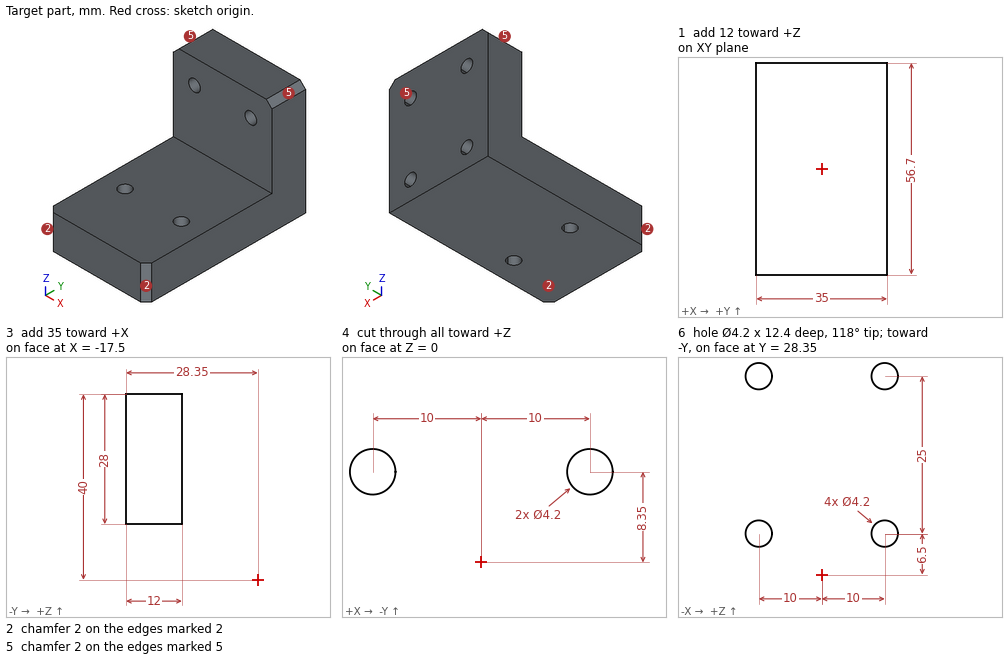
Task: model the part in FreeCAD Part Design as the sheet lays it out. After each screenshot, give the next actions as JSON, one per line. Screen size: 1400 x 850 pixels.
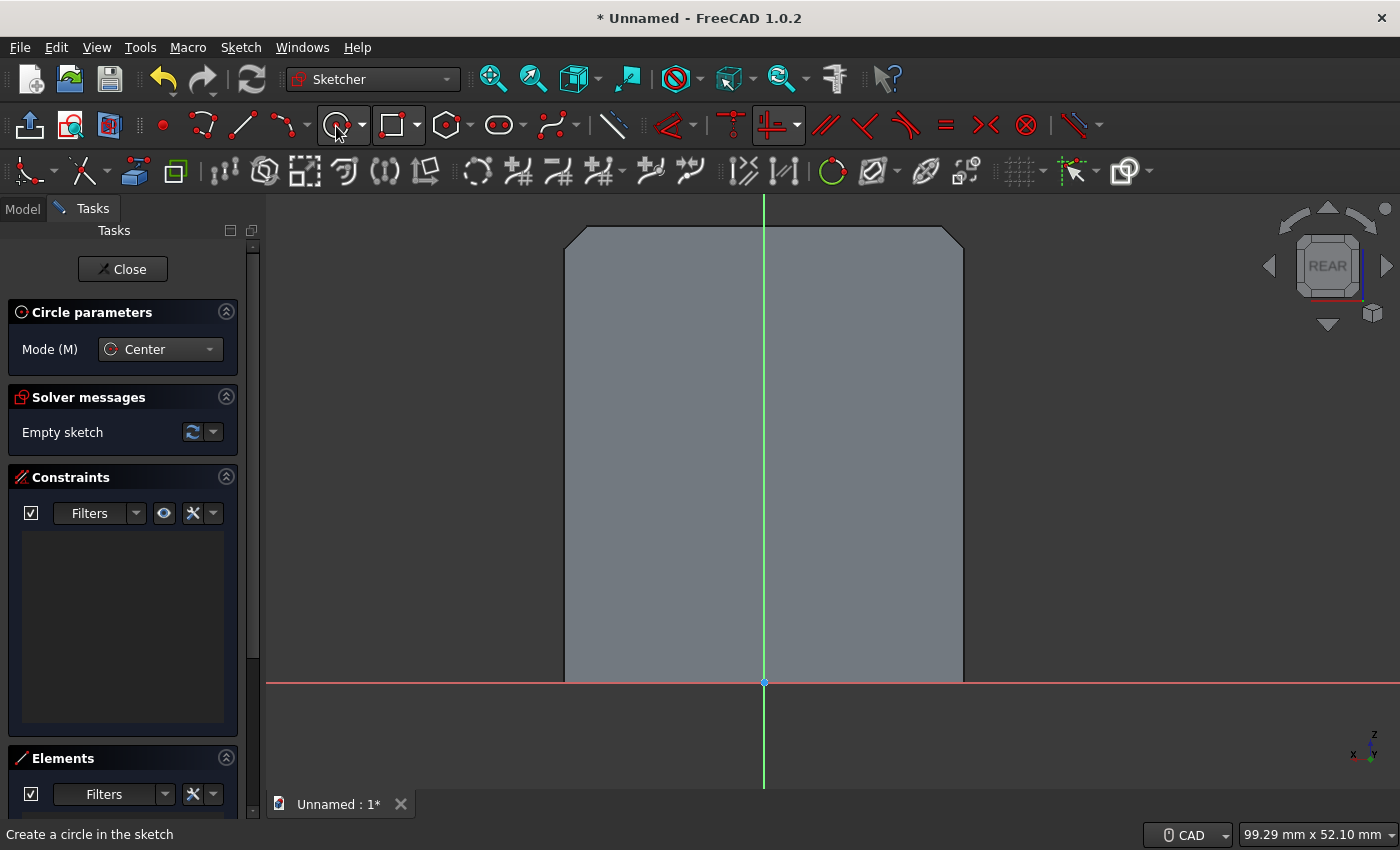
{"action": "left_click", "coordinate": [879, 609]}
{"action": "left_click", "coordinate": [896, 592]}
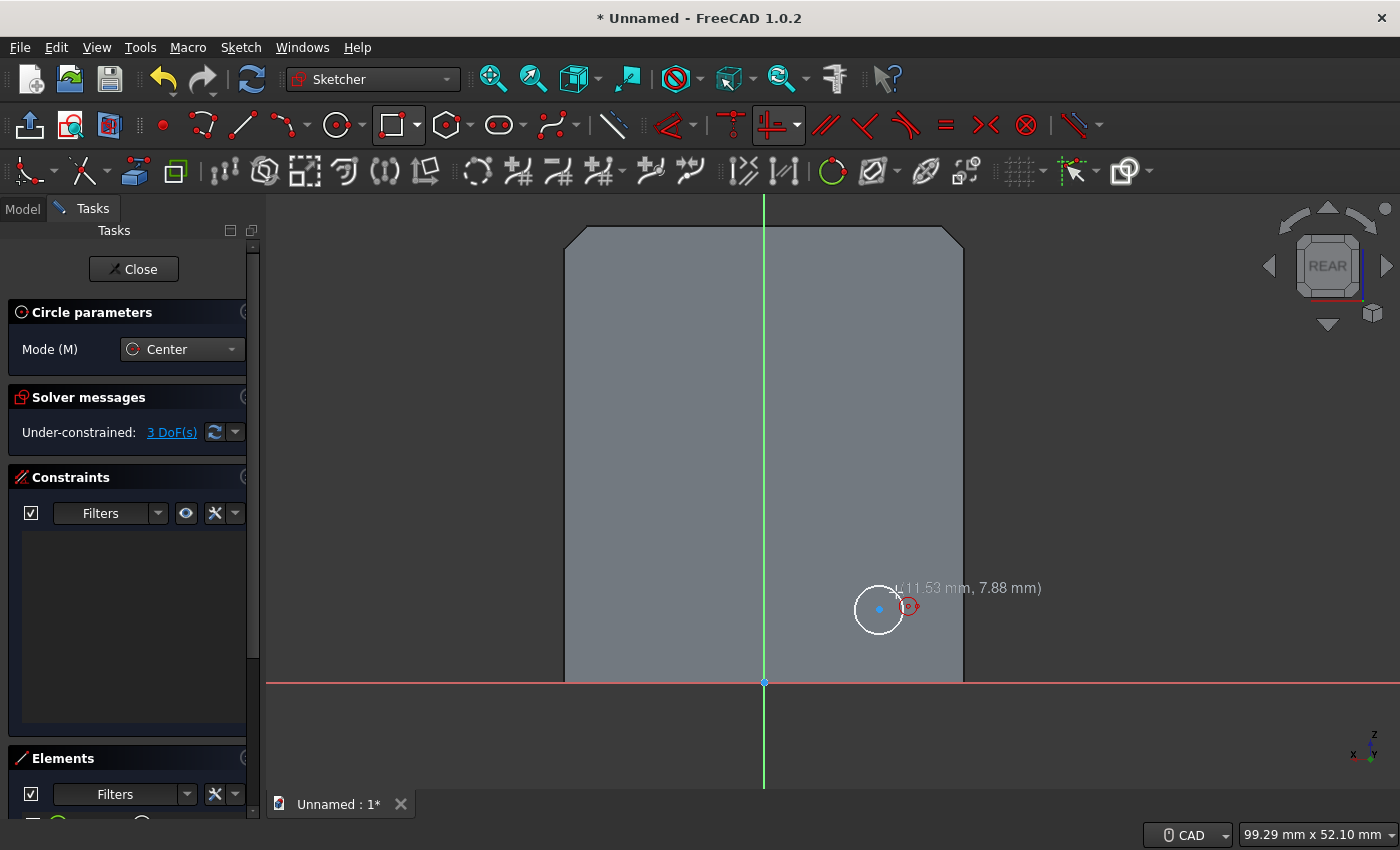
{"action": "left_click", "coordinate": [650, 609]}
{"action": "left_click", "coordinate": [667, 592]}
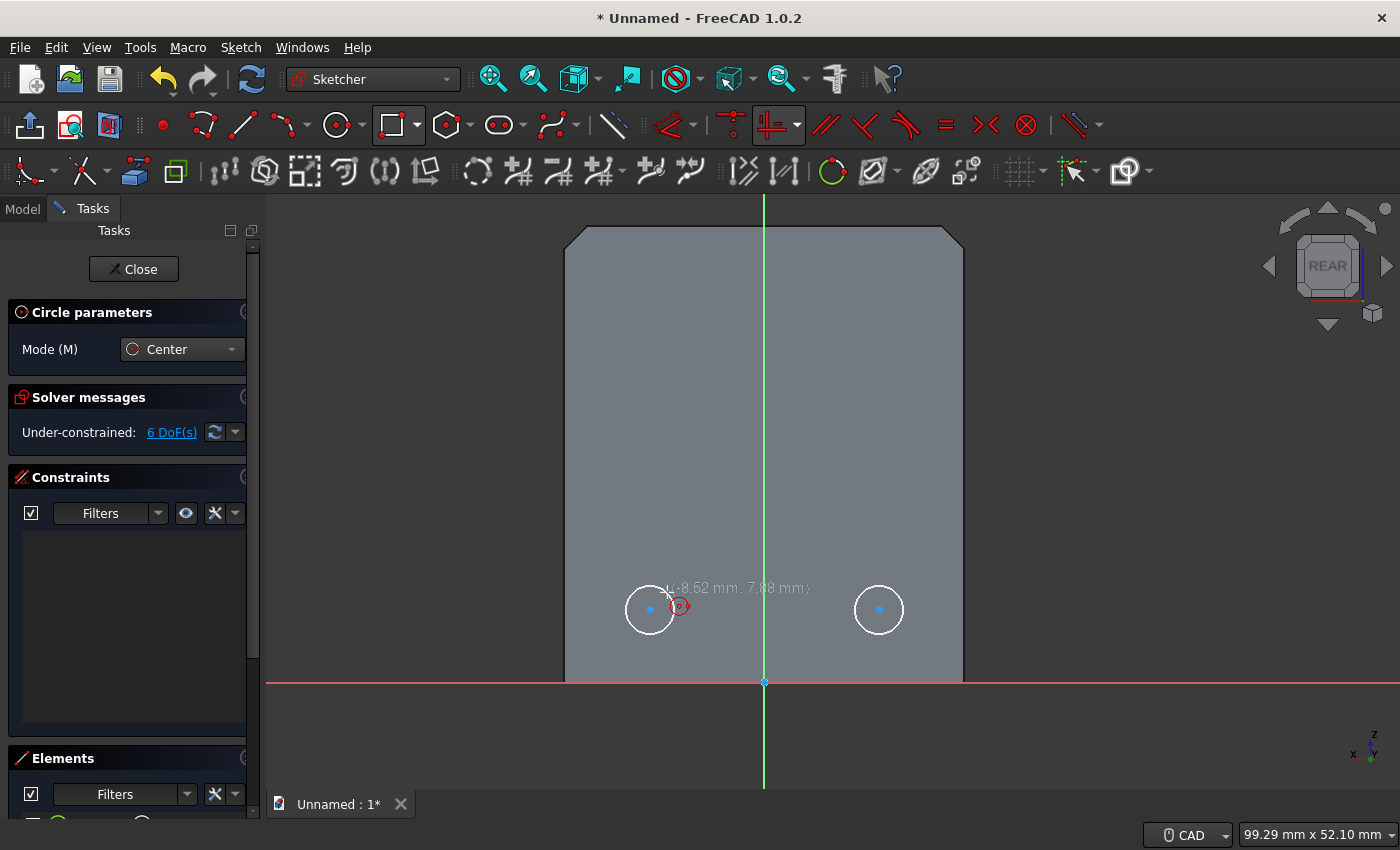
{"action": "left_click", "coordinate": [879, 323]}
{"action": "left_click", "coordinate": [896, 306]}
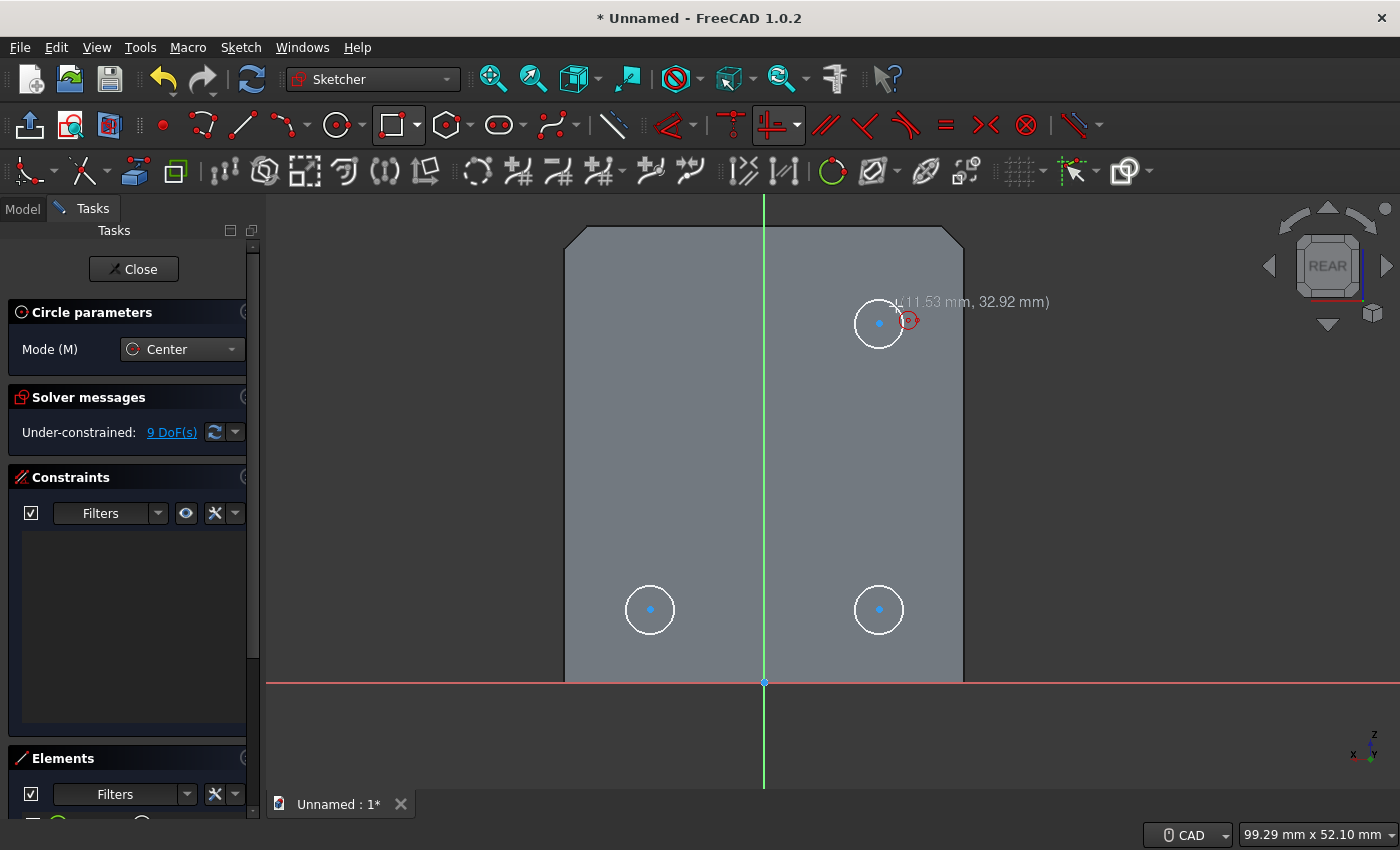
{"action": "left_click", "coordinate": [650, 323]}
{"action": "left_click", "coordinate": [667, 306]}
{"action": "key", "text": "Escape"}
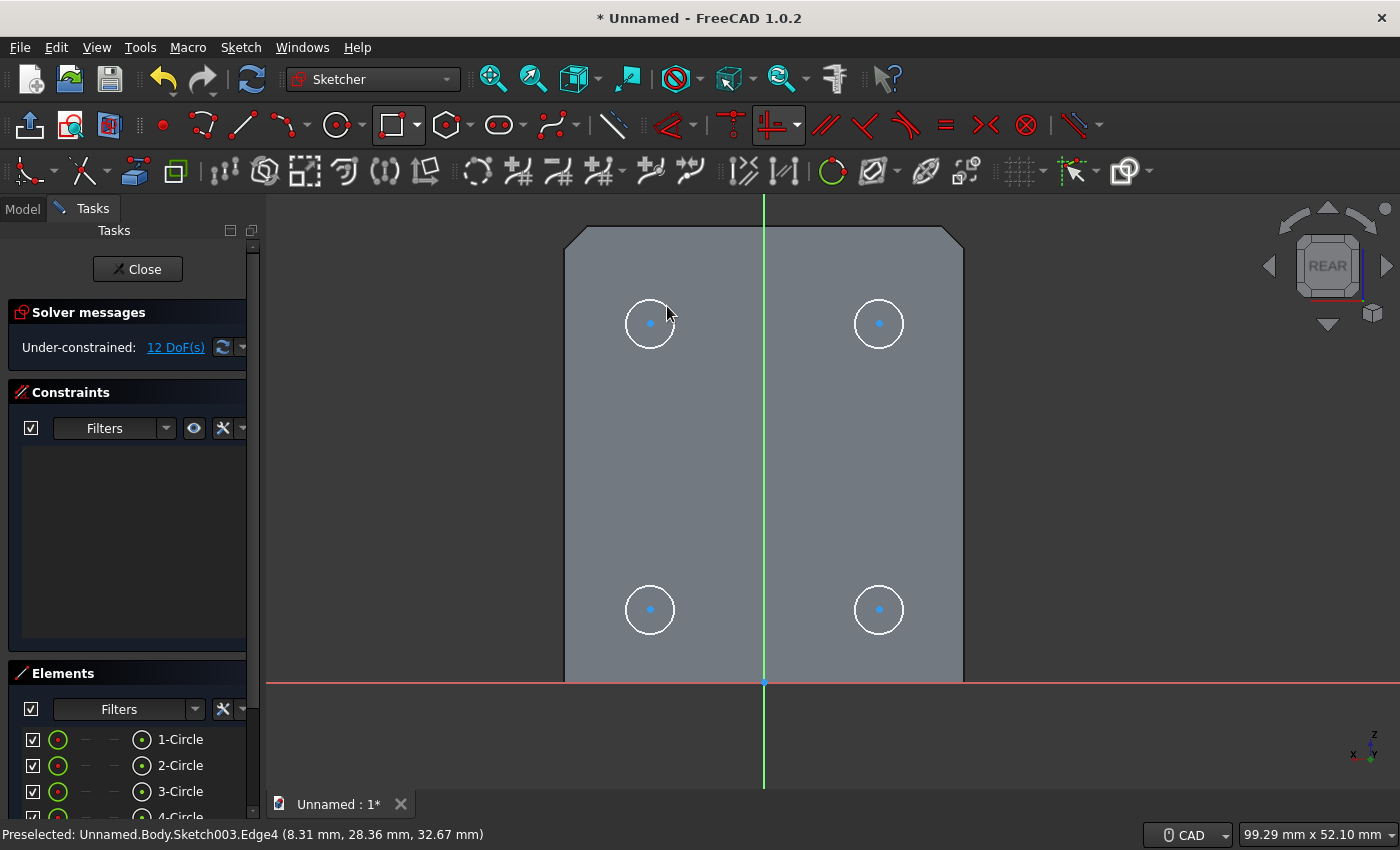
{"action": "left_click", "coordinate": [896, 593]}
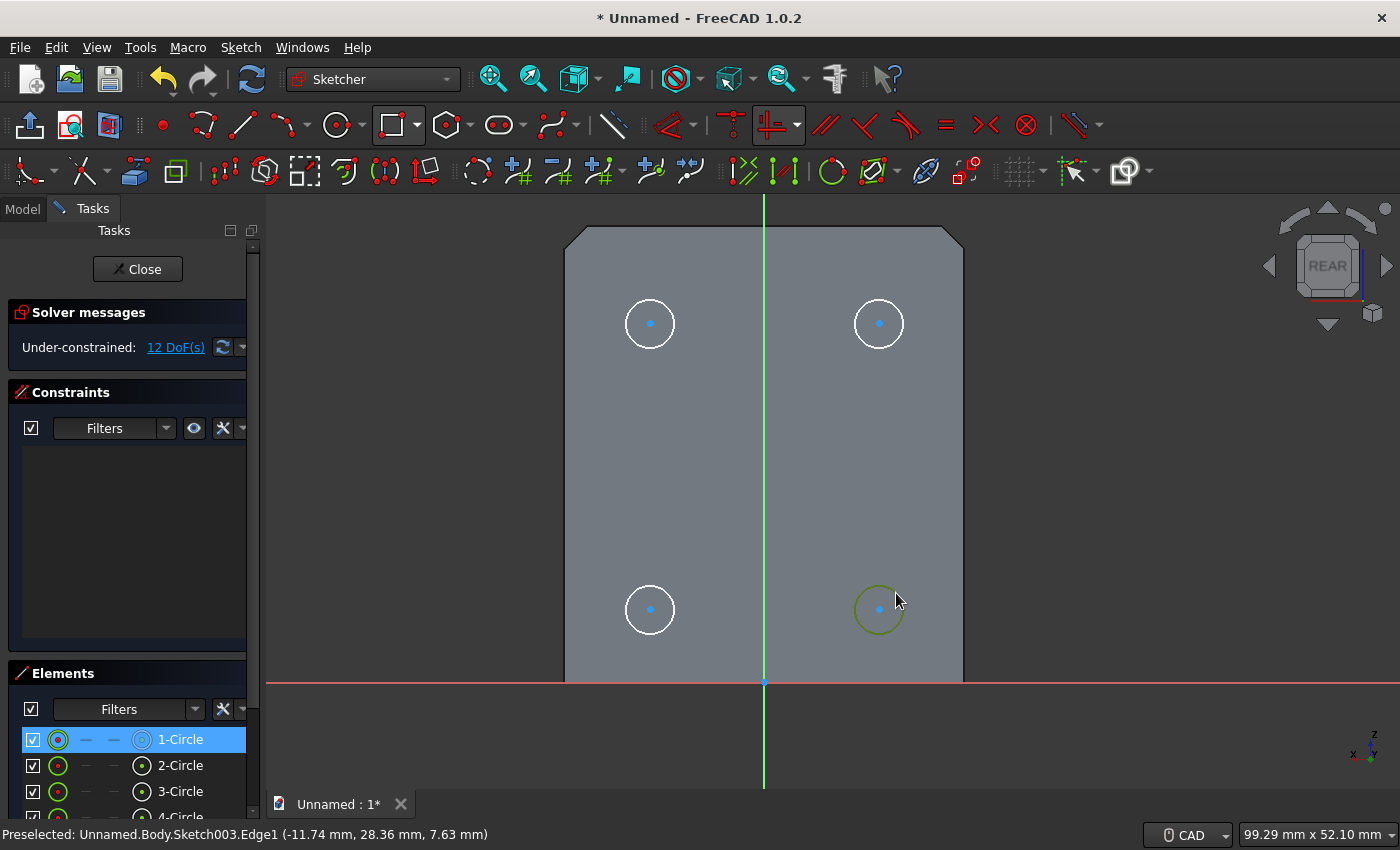
{"action": "left_click", "coordinate": [667, 593]}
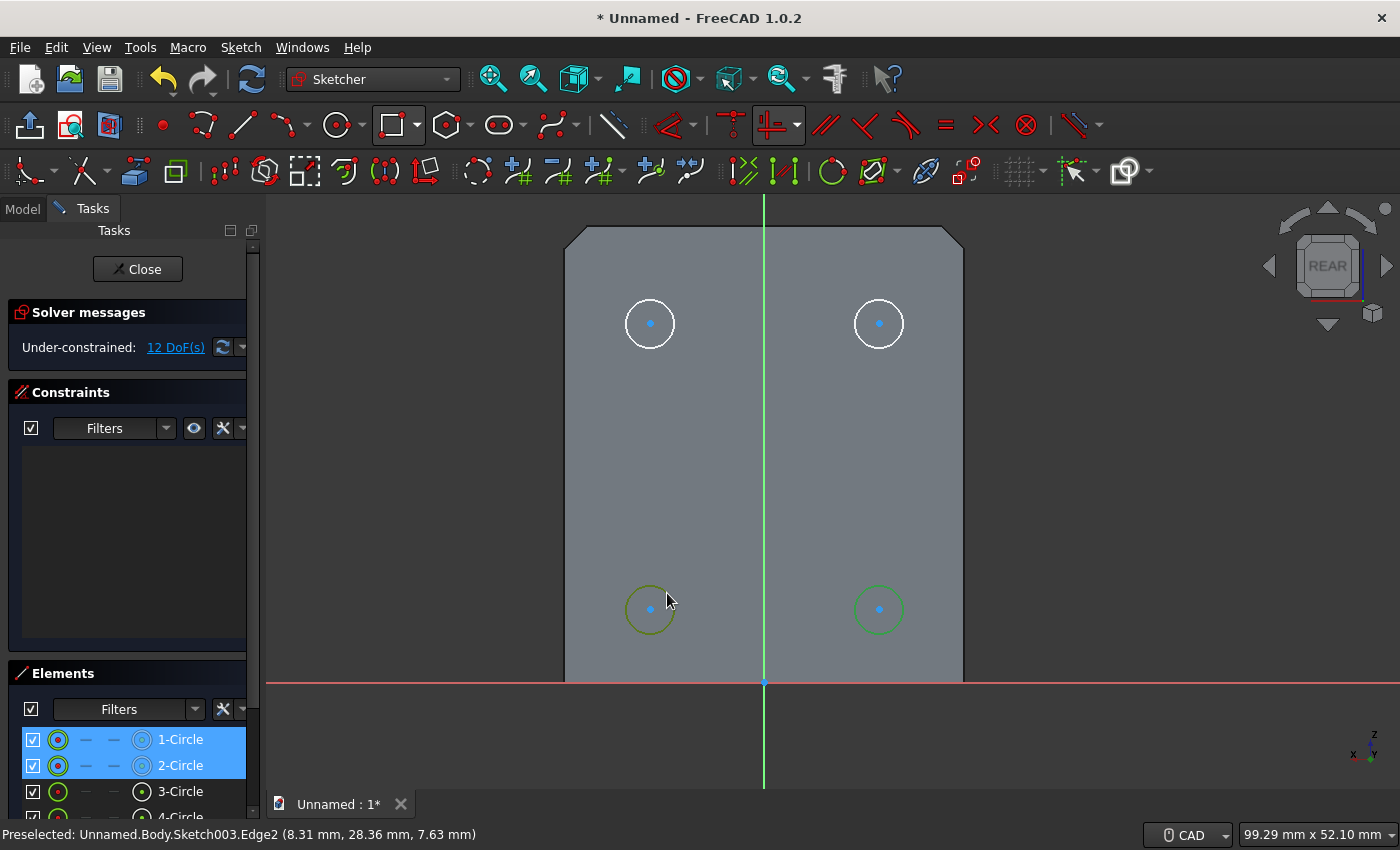
{"action": "left_click", "coordinate": [896, 307]}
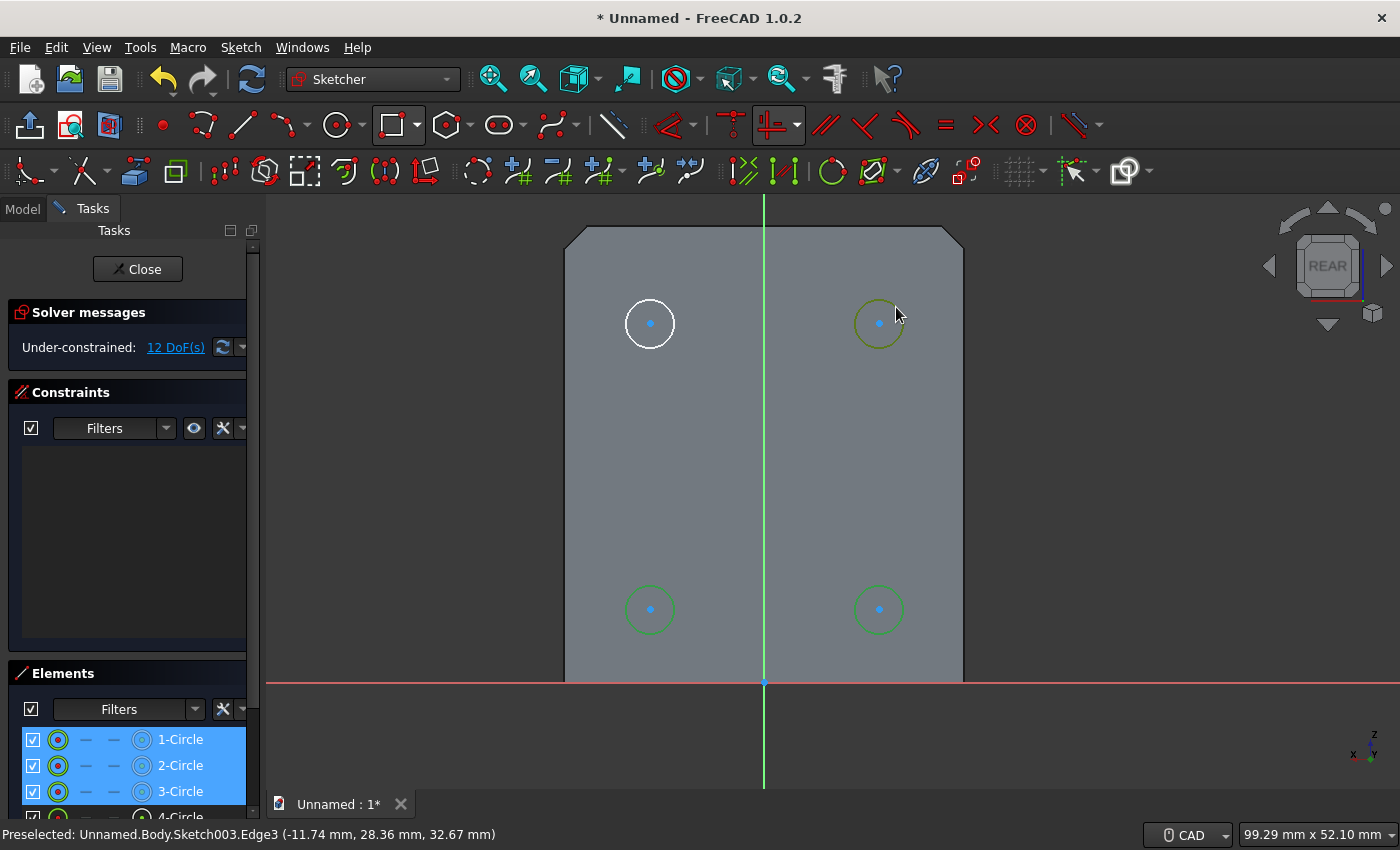
{"action": "left_click", "coordinate": [667, 307]}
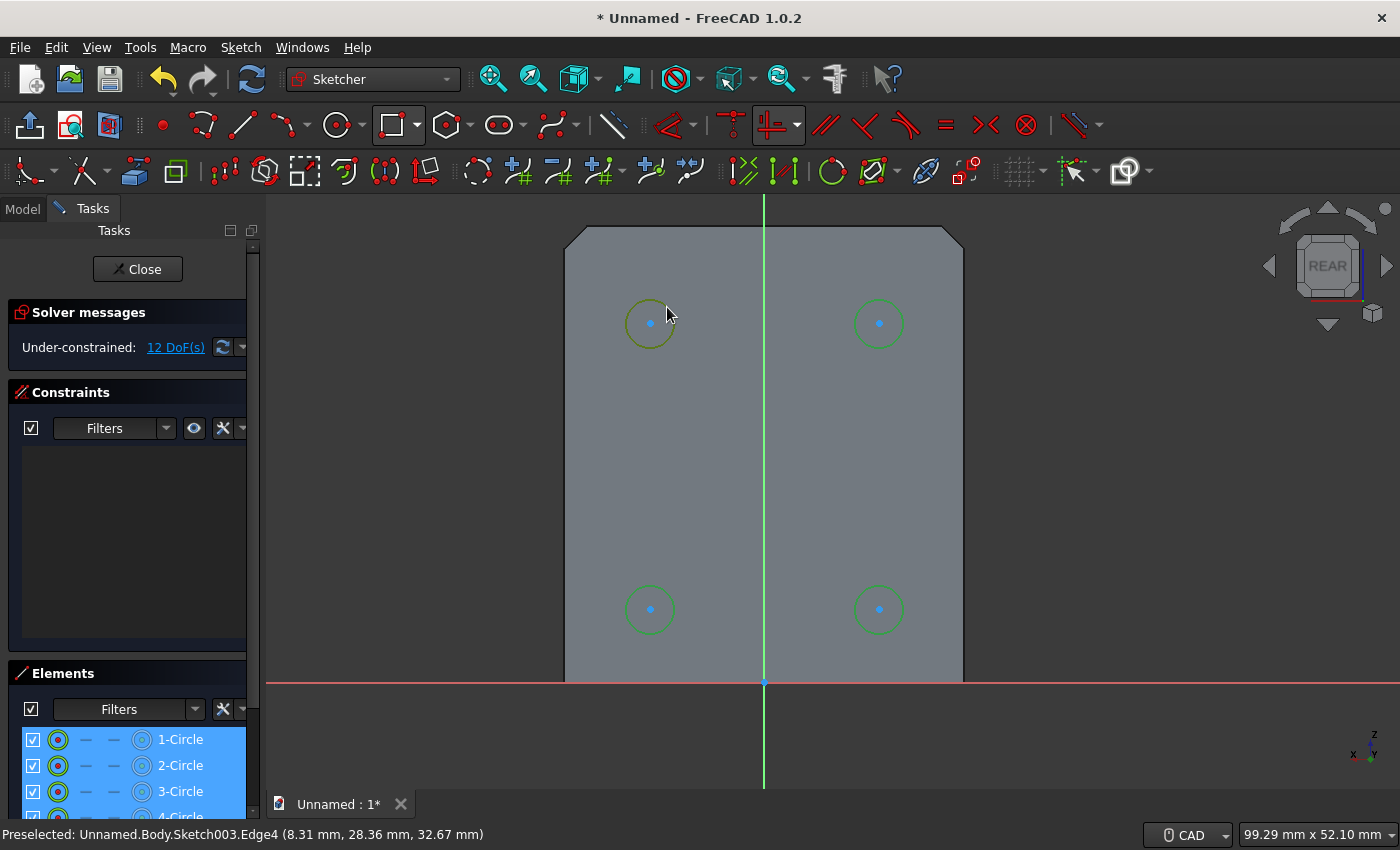
{"action": "left_click", "coordinate": [946, 126]}